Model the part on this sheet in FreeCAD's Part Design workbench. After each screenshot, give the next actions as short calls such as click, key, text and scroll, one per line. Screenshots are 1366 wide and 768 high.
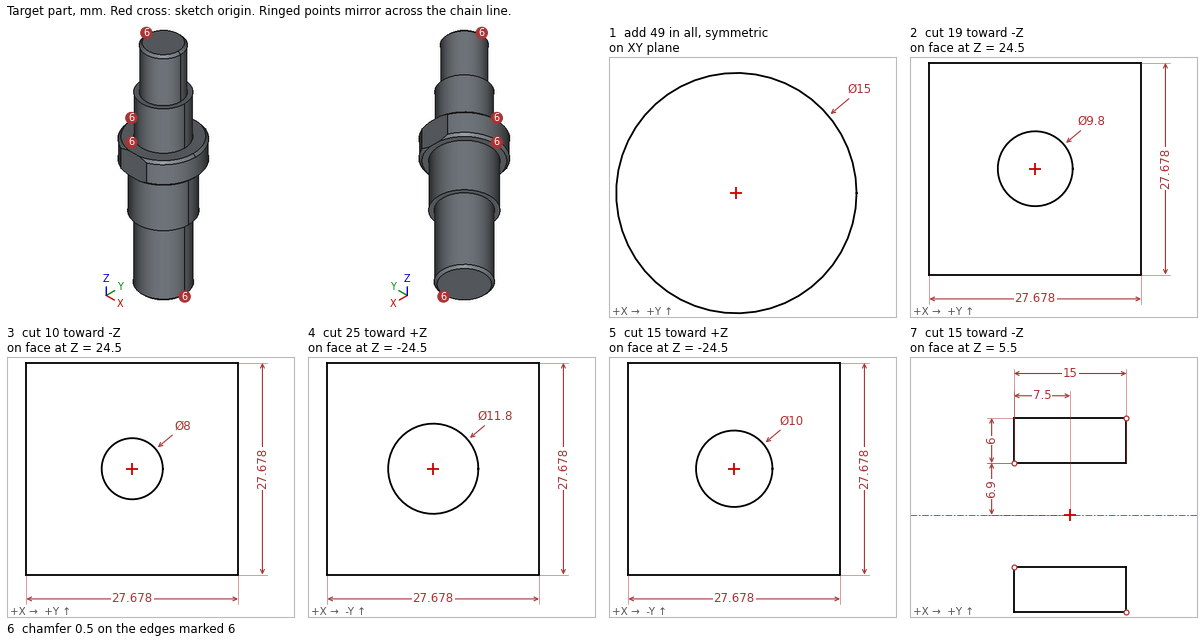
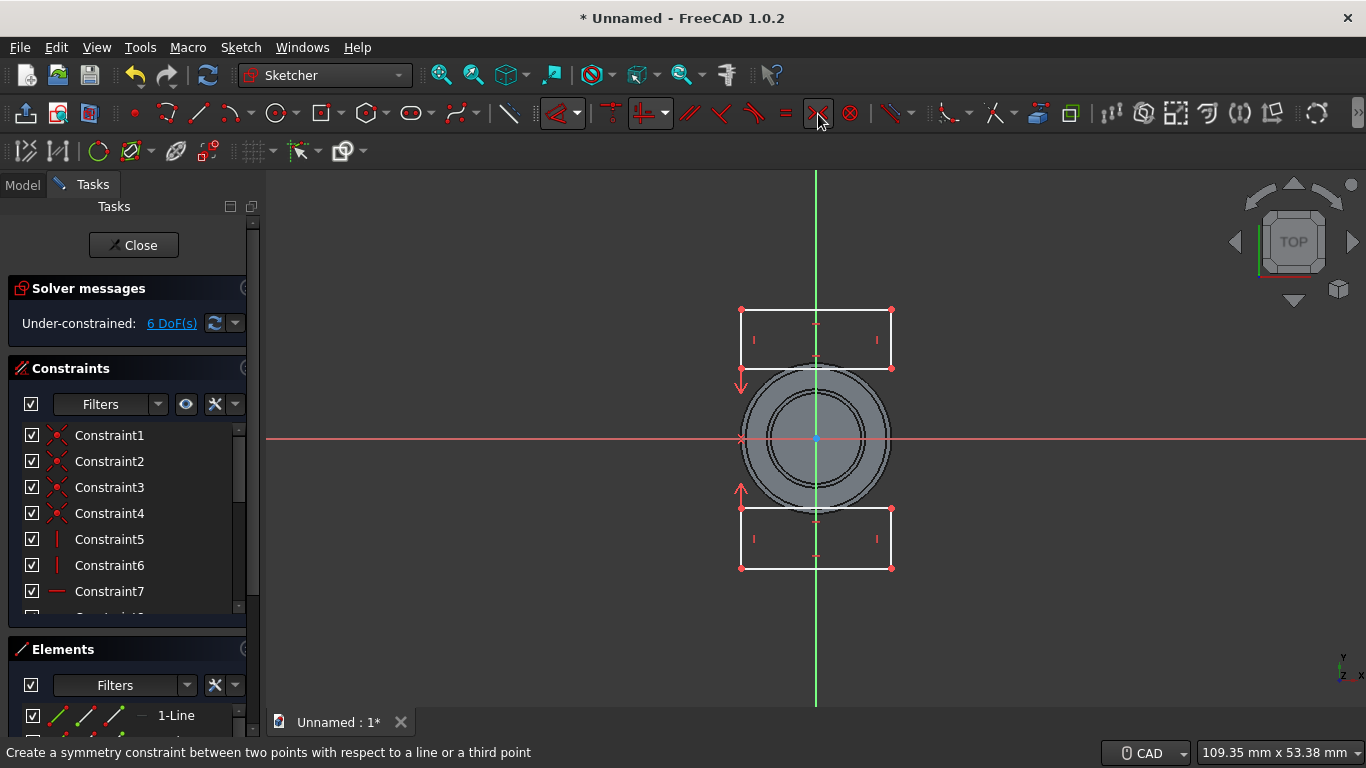
click(891, 310)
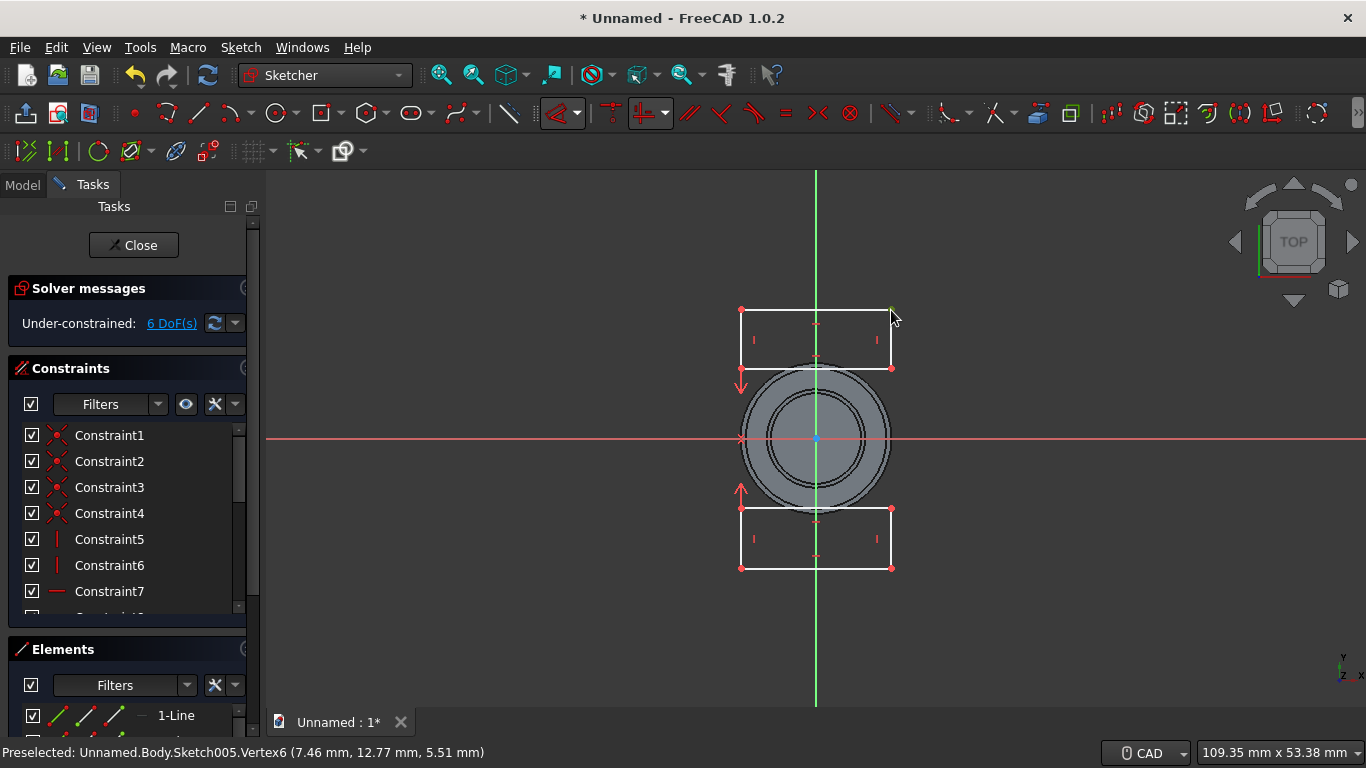
click(891, 569)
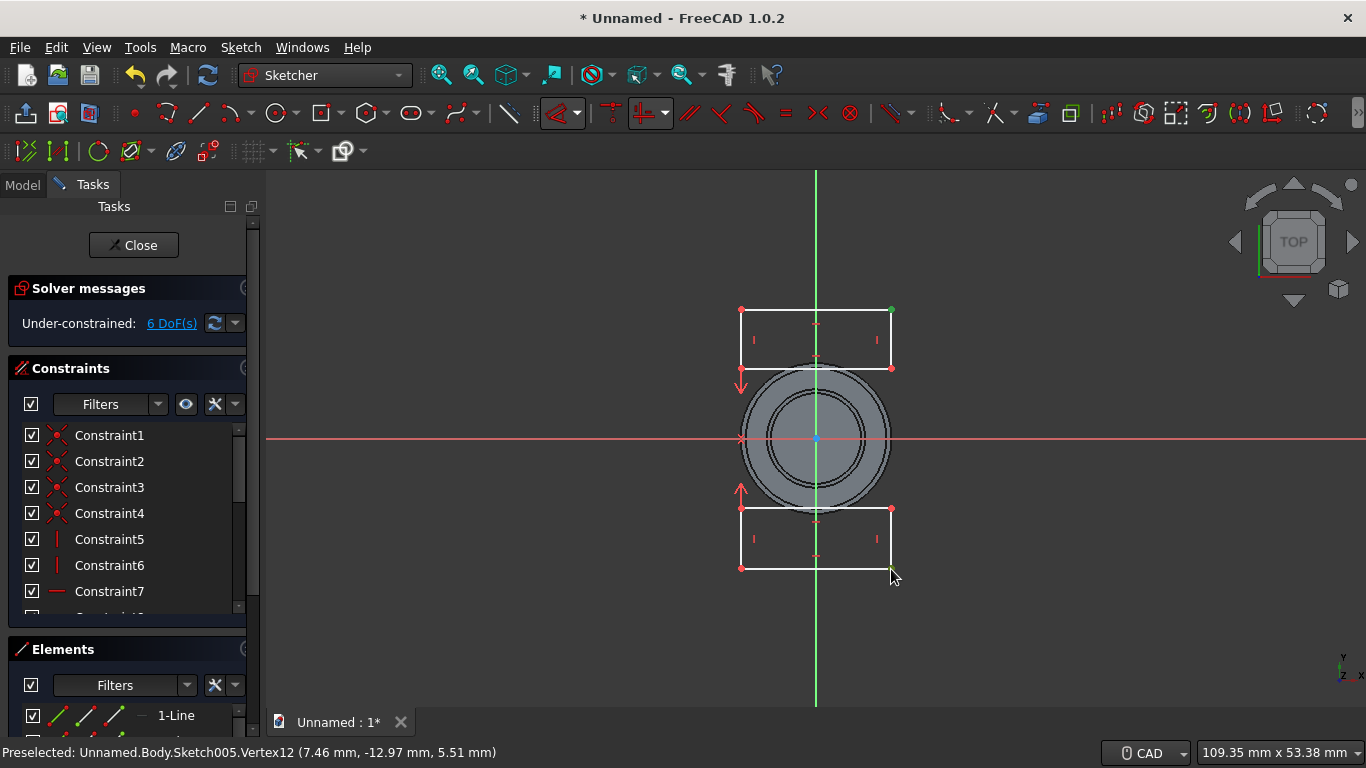
click(359, 439)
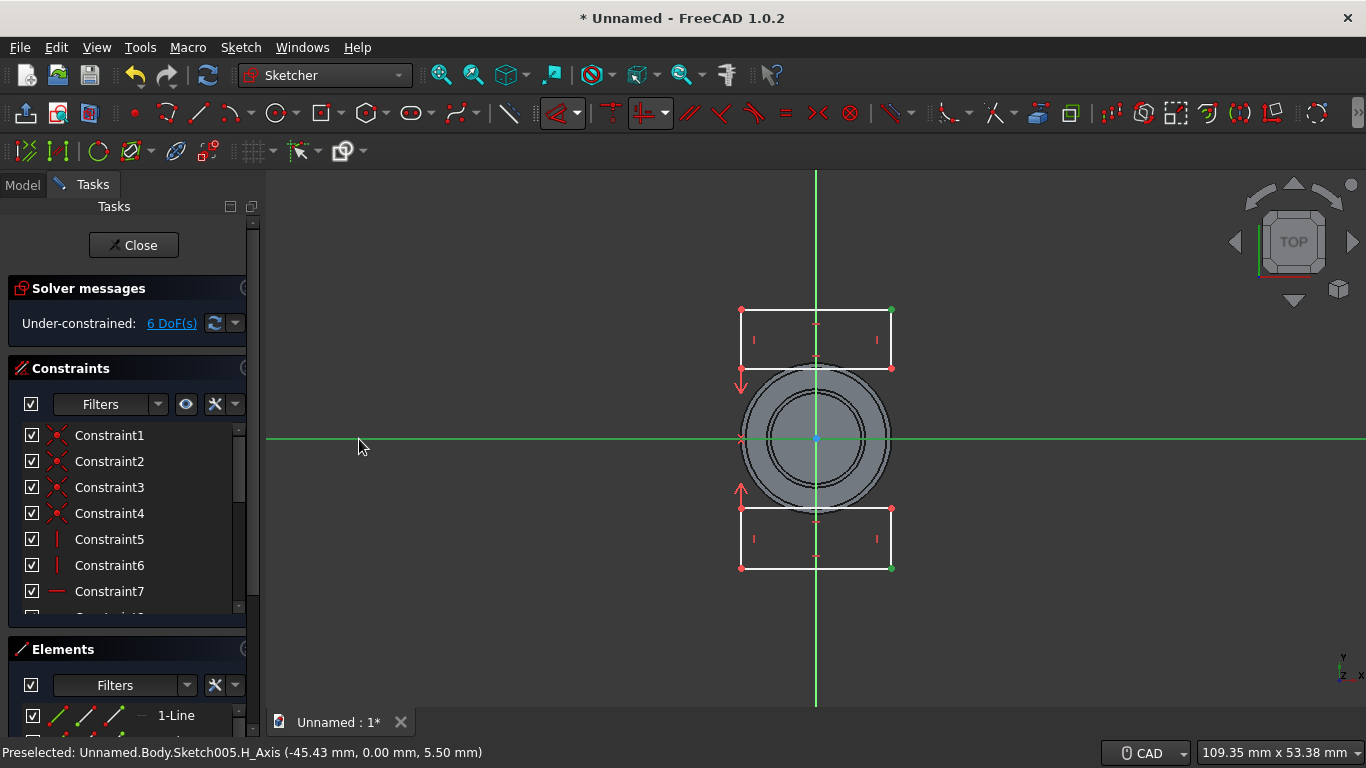
click(818, 114)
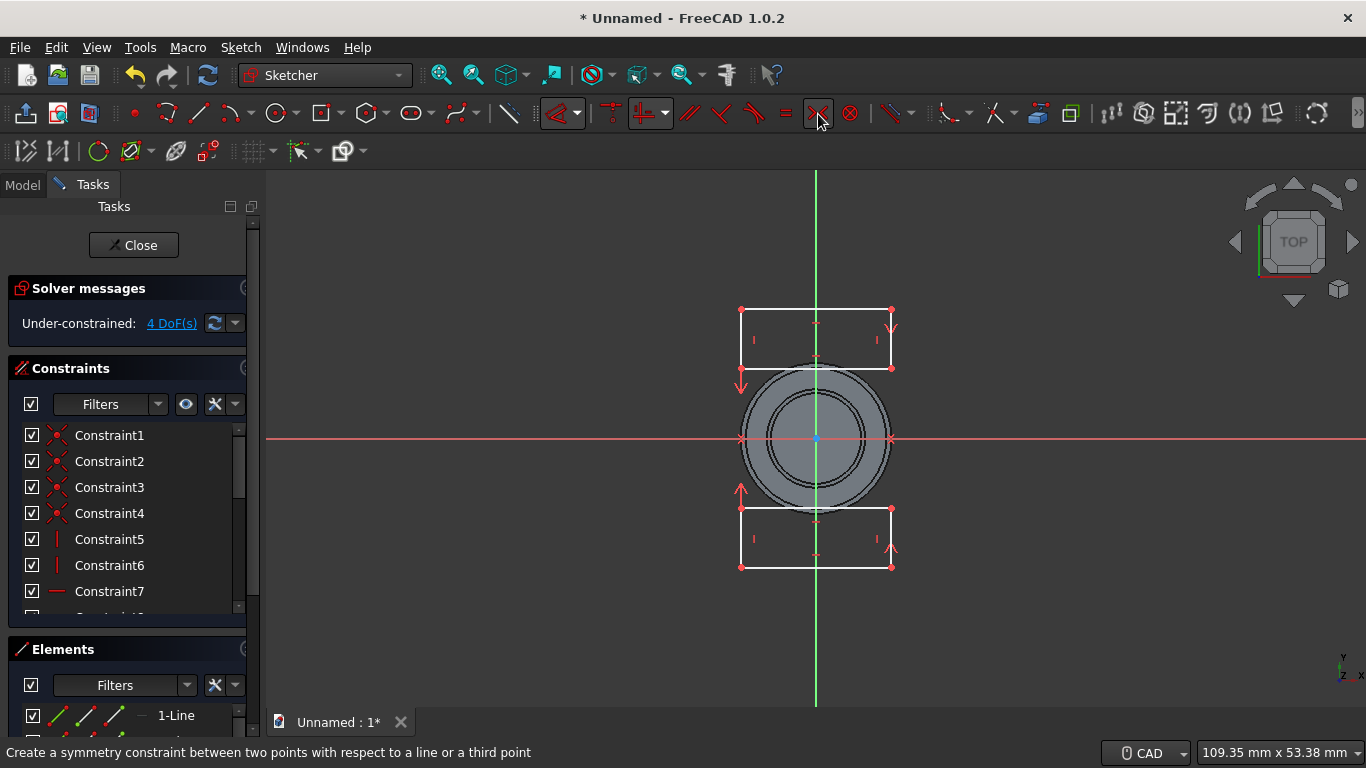
click(741, 327)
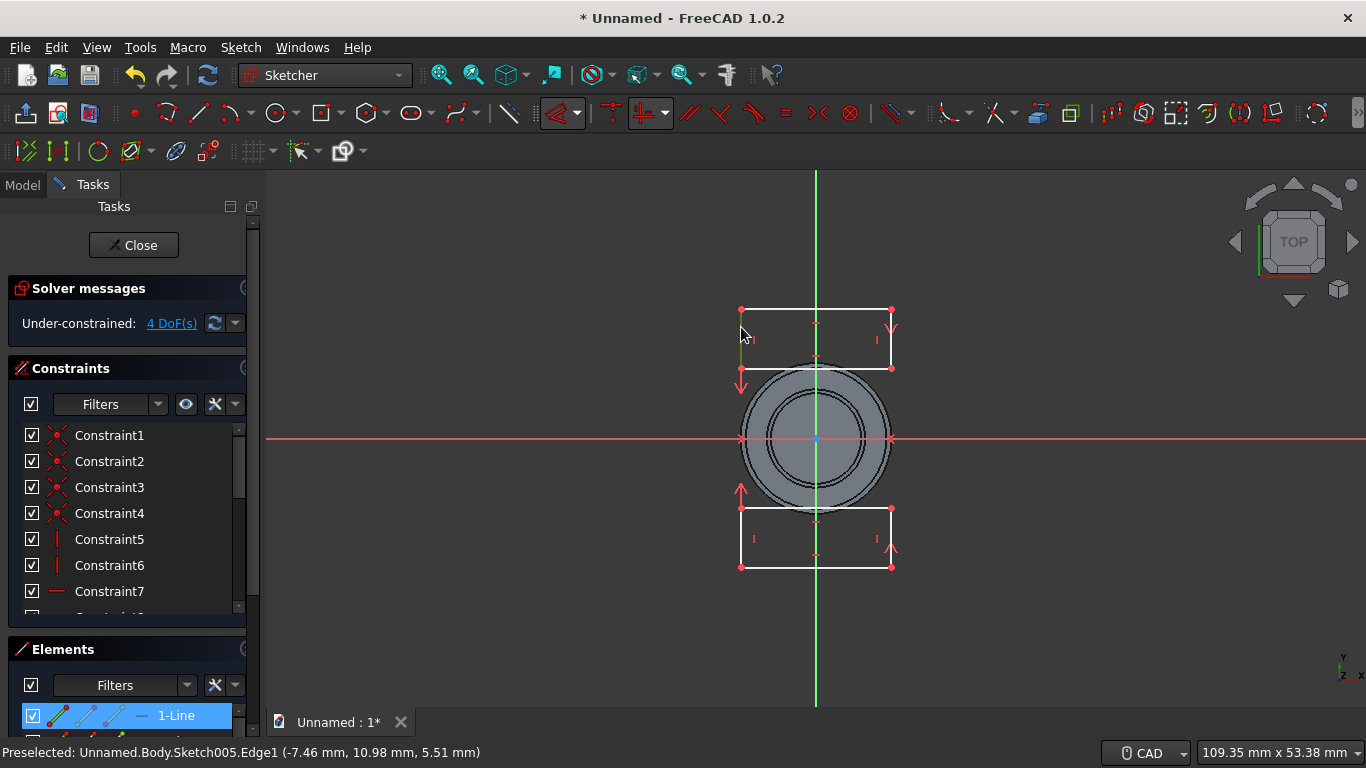
key(i)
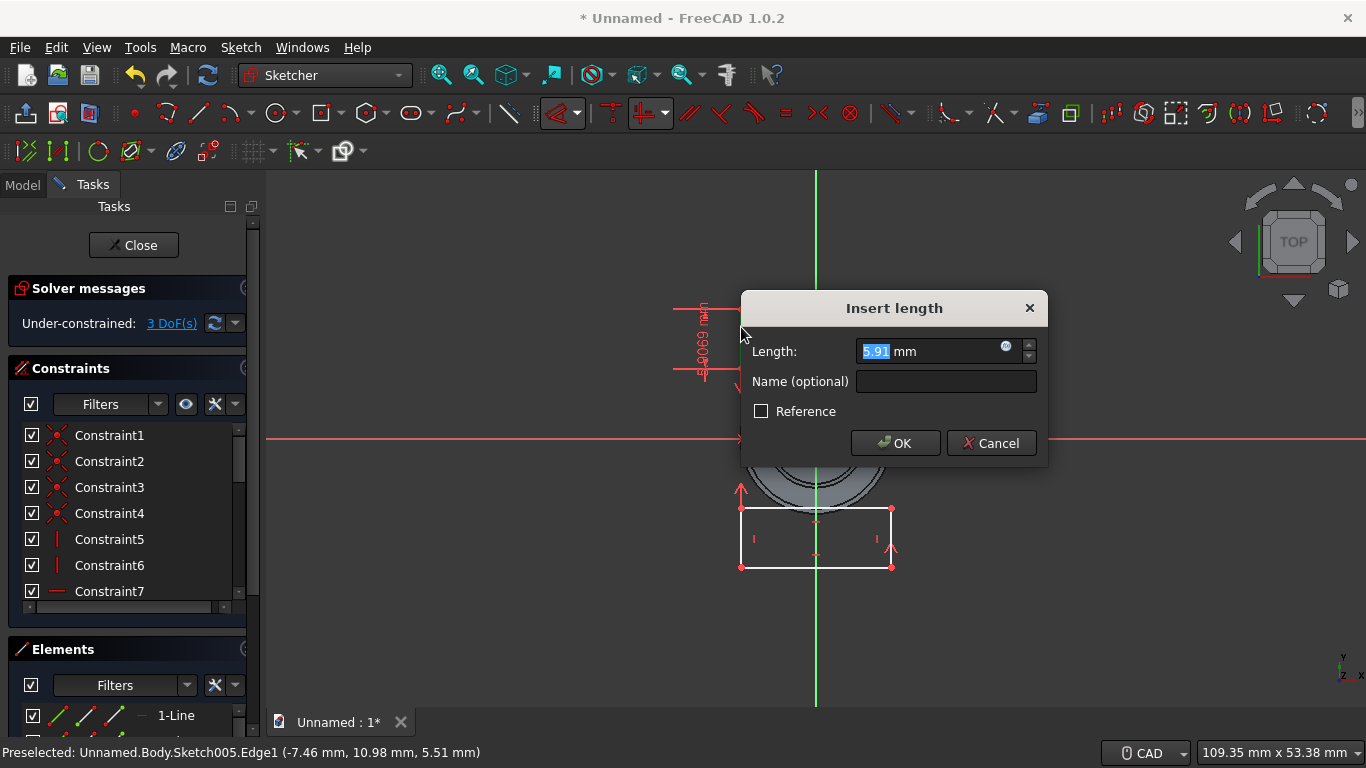
text(6)
key(Return)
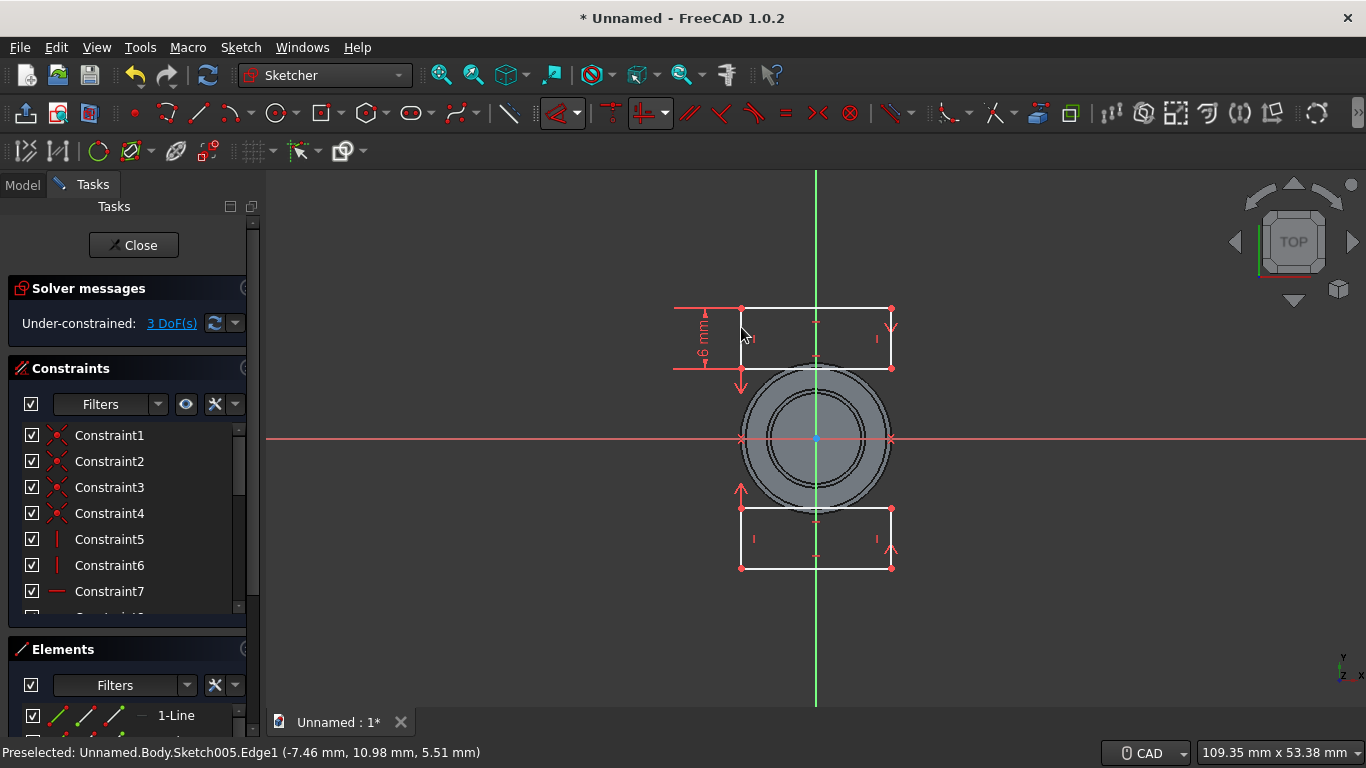
click(786, 369)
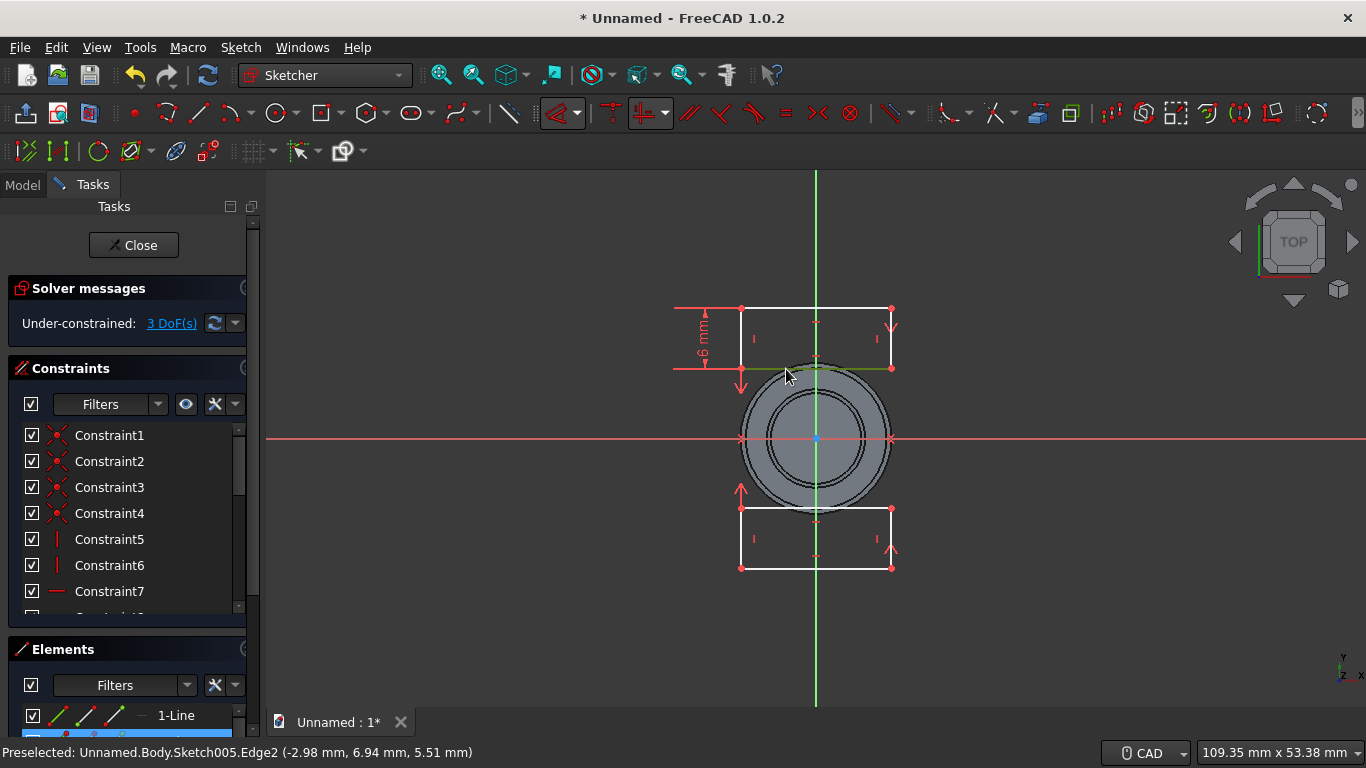
click(580, 114)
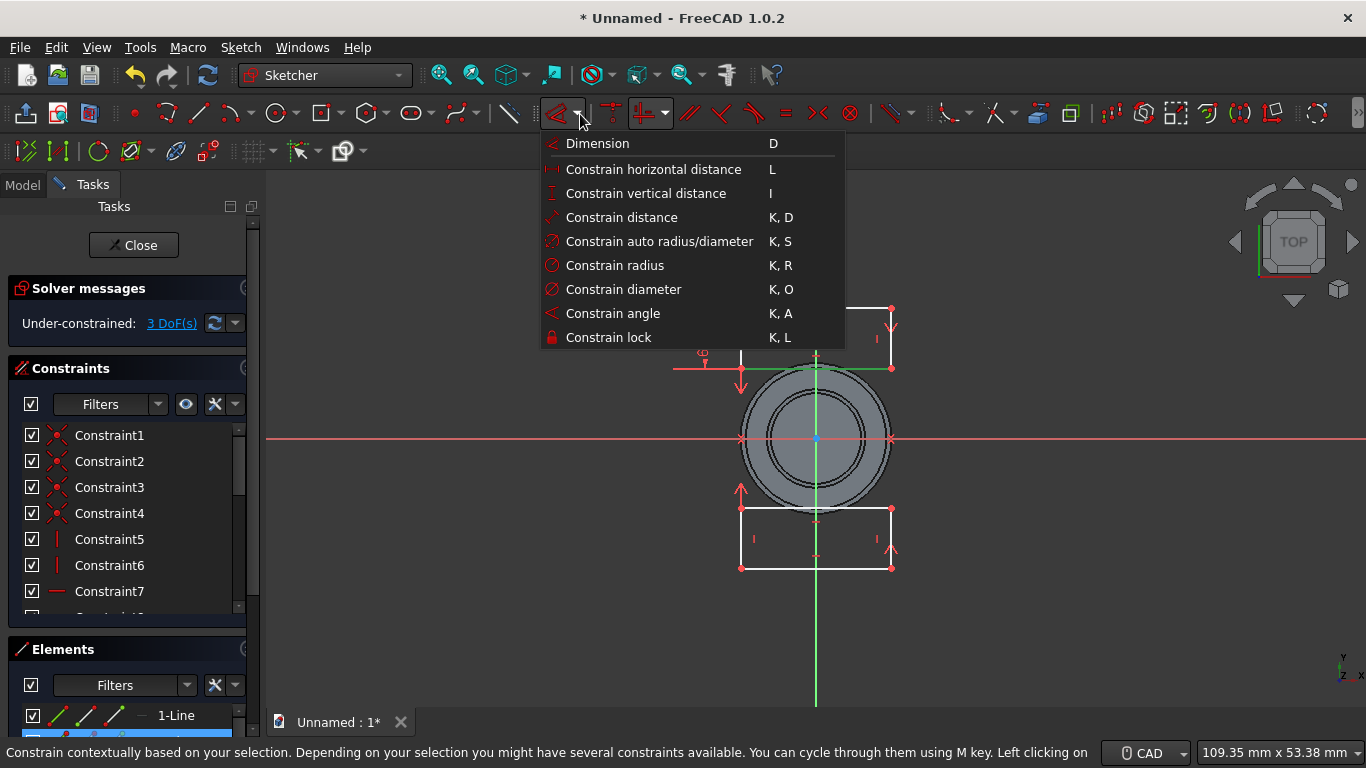
click(693, 169)